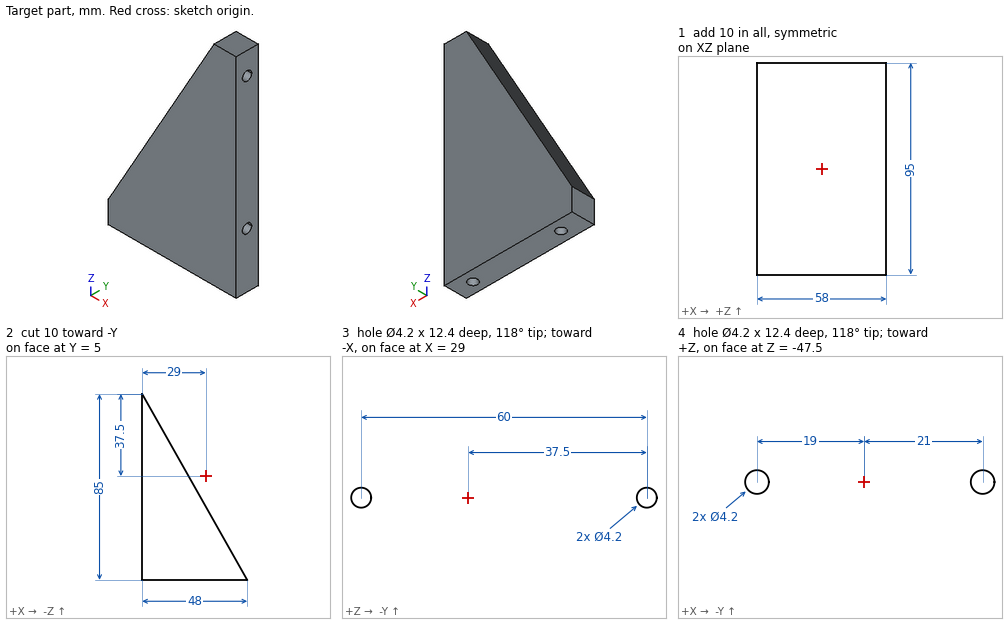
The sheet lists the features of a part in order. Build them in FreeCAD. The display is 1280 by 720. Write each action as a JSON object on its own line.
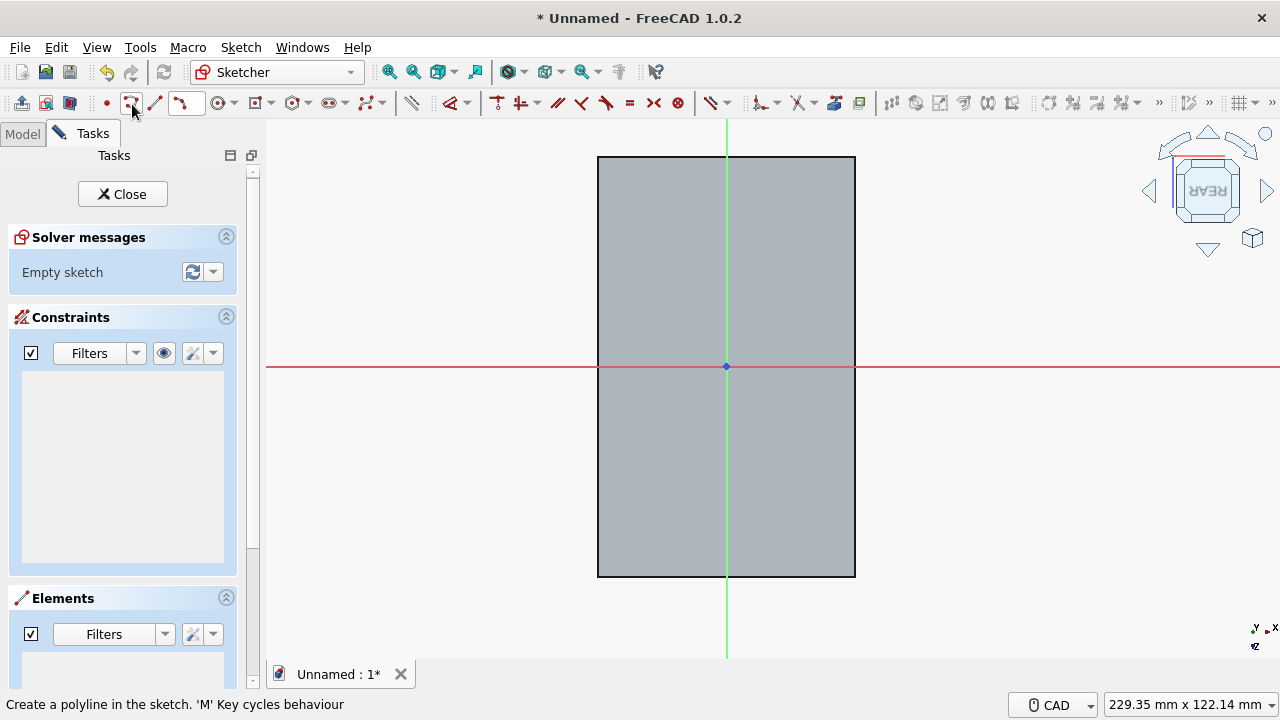
{"action": "left_click", "coordinate": [598, 201]}
{"action": "left_click", "coordinate": [598, 577]}
{"action": "left_click", "coordinate": [811, 577]}
{"action": "left_click", "coordinate": [598, 202]}
{"action": "key", "text": "Escape"}
{"action": "key", "text": "Escape"}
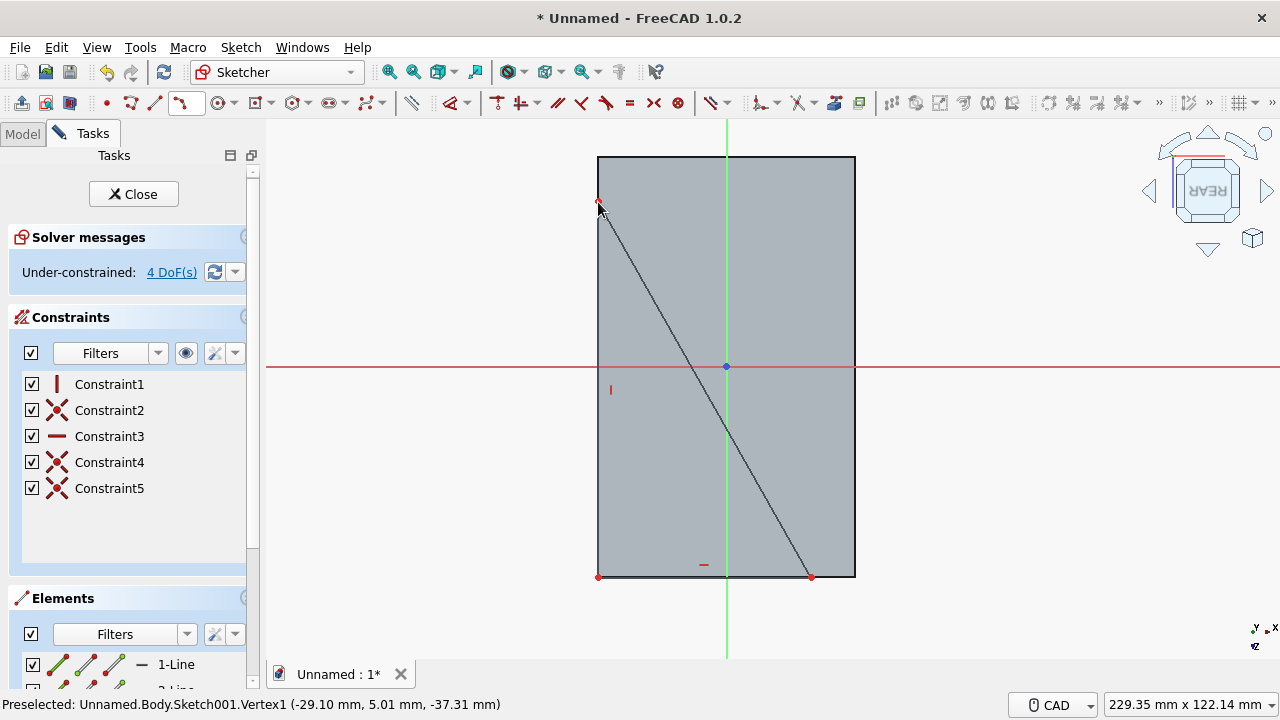
{"action": "left_click", "coordinate": [450, 104]}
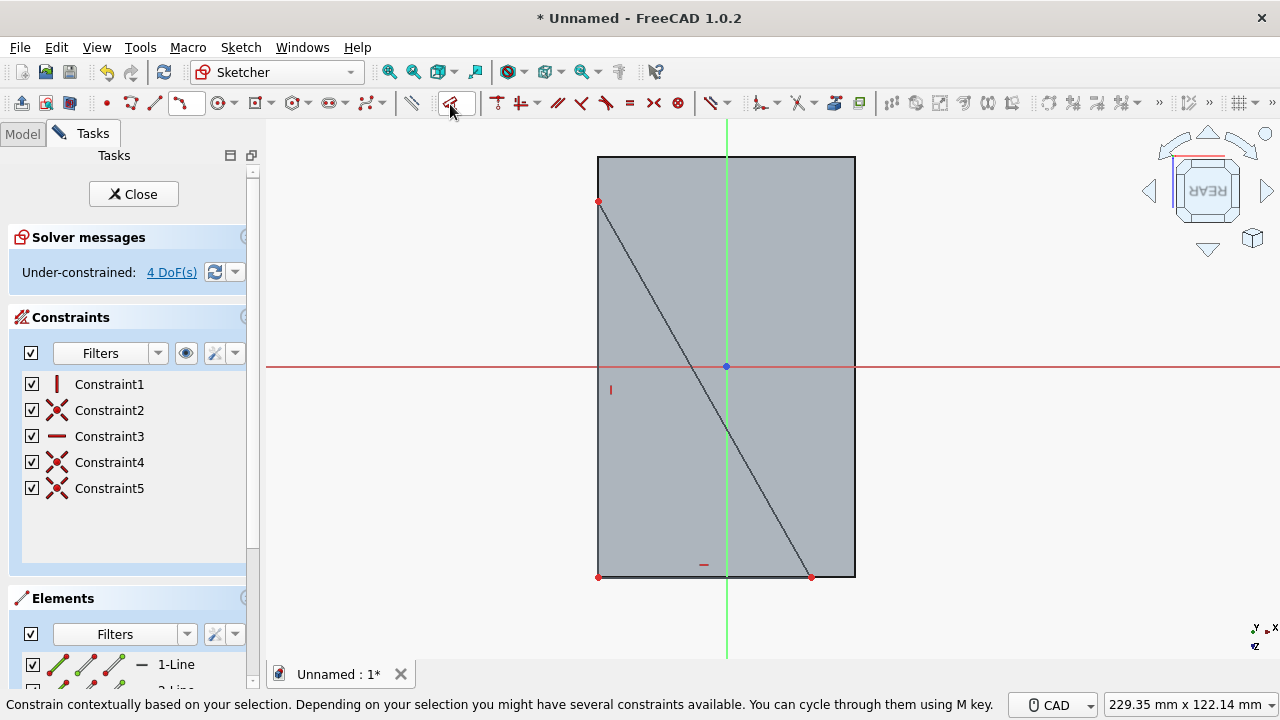
{"action": "left_click", "coordinate": [598, 315]}
{"action": "left_click", "coordinate": [564, 390]}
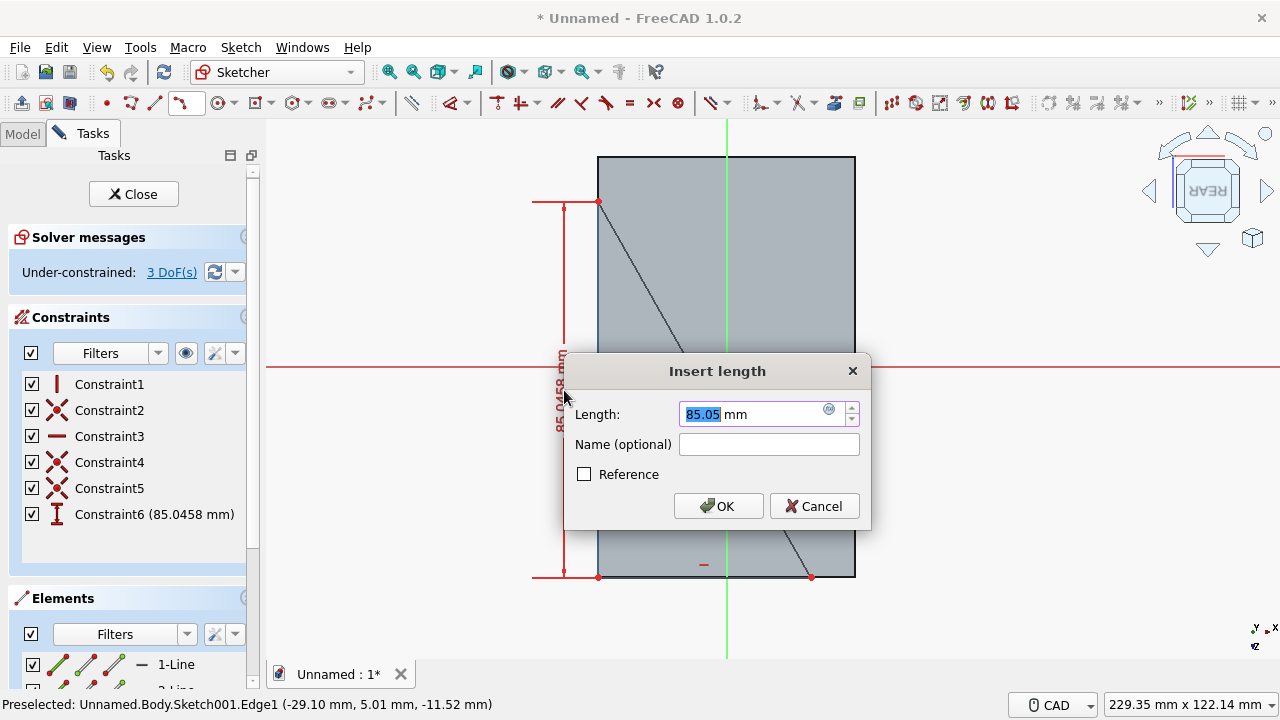
{"action": "type", "text": "85"}
{"action": "key", "text": "Return"}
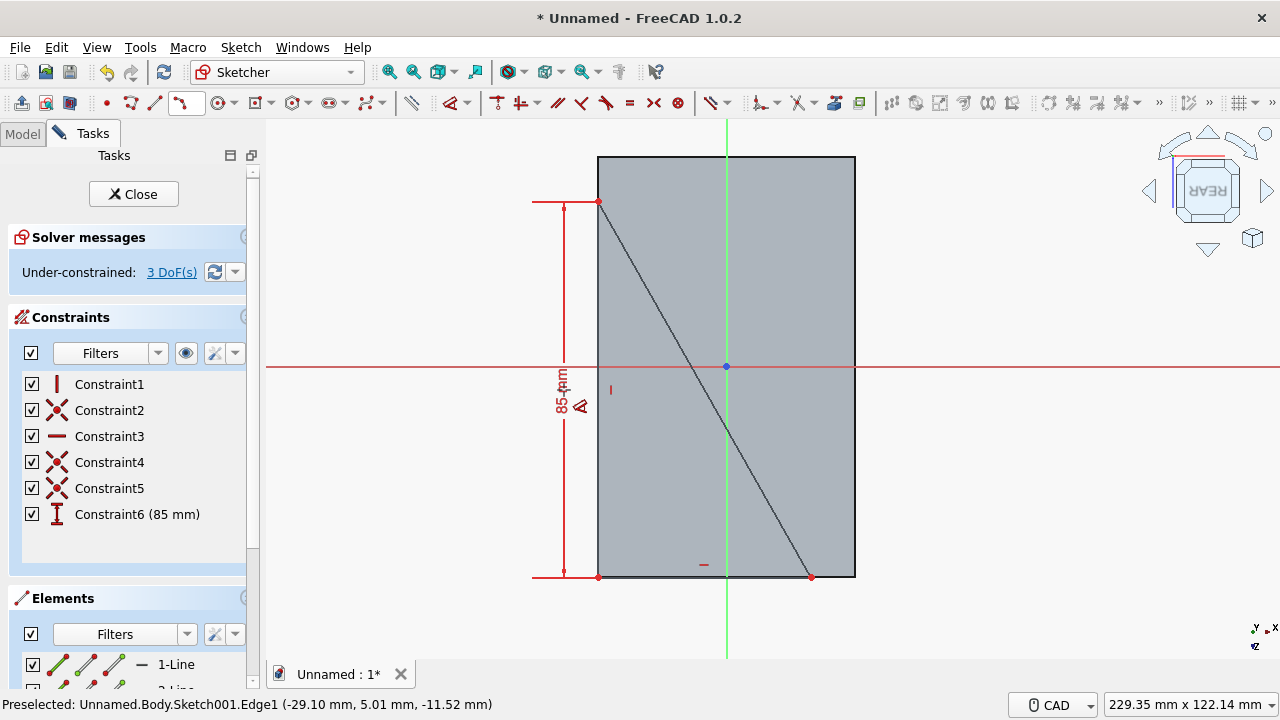
{"action": "left_click", "coordinate": [662, 578]}
{"action": "left_click", "coordinate": [705, 612]}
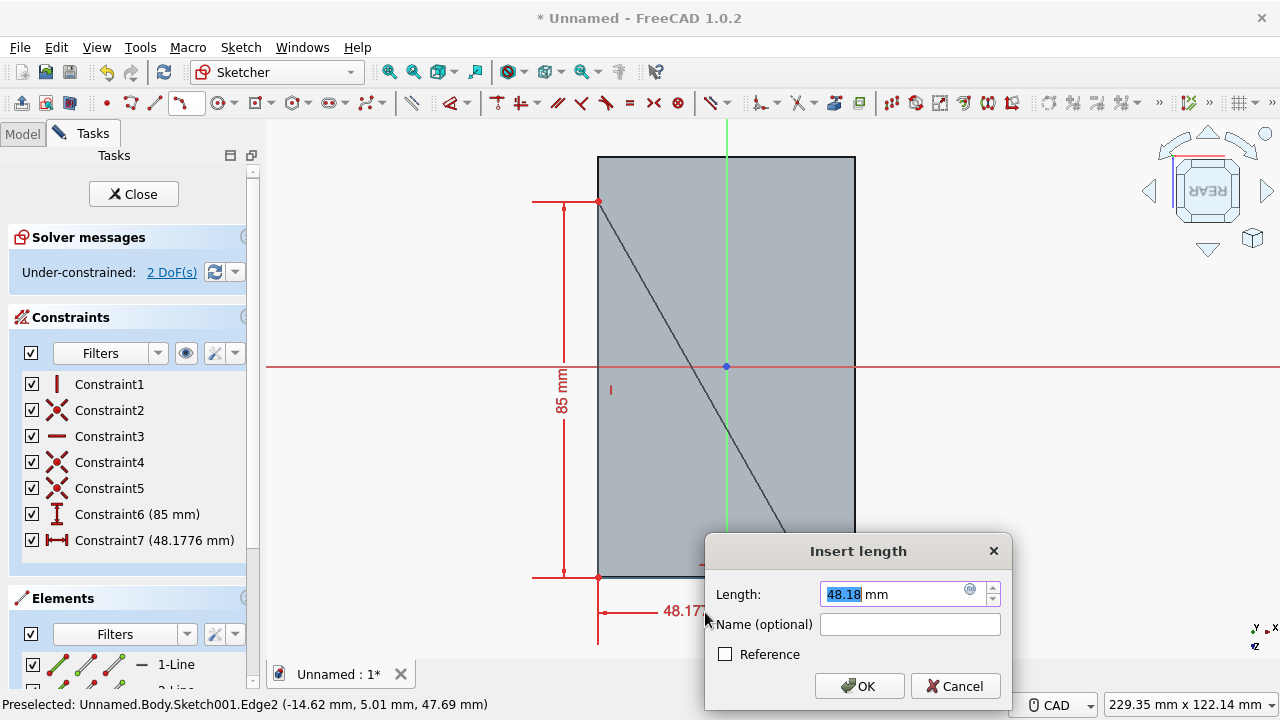
{"action": "type", "text": "48"}
{"action": "key", "text": "Return"}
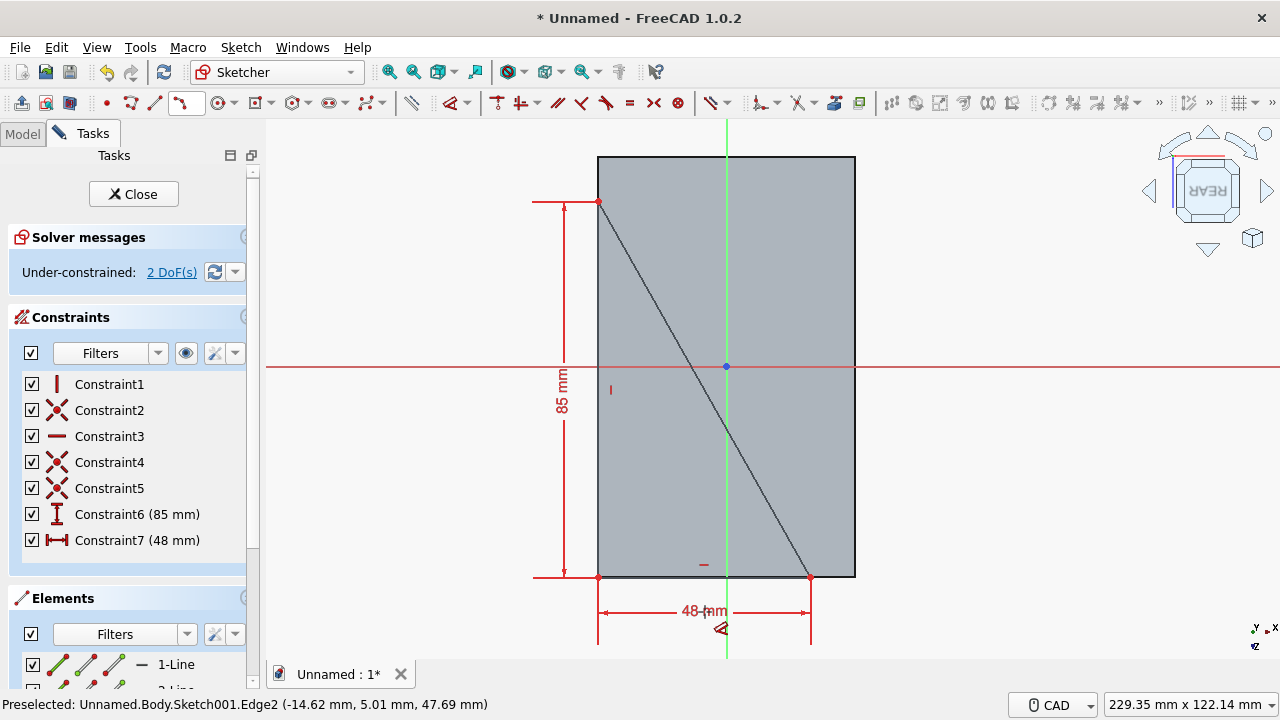
{"action": "left_click", "coordinate": [598, 202]}
{"action": "left_click", "coordinate": [662, 168]}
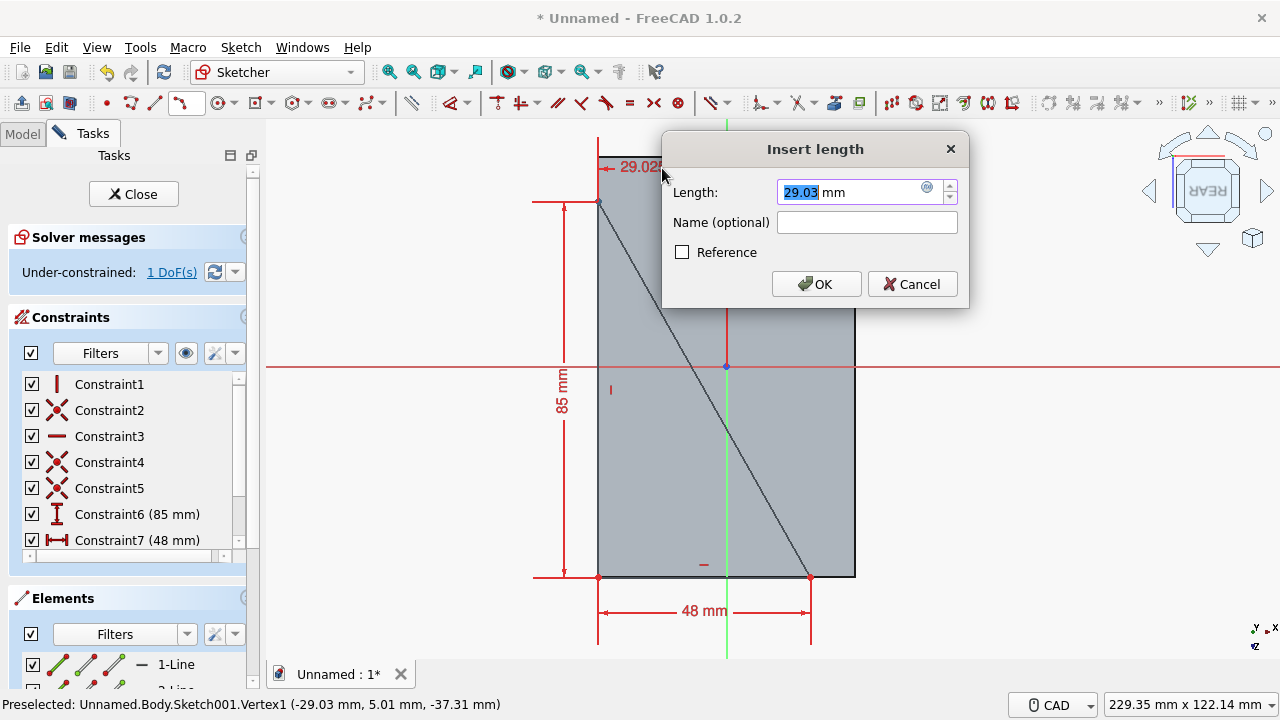
{"action": "type", "text": "29"}
{"action": "key", "text": "Return"}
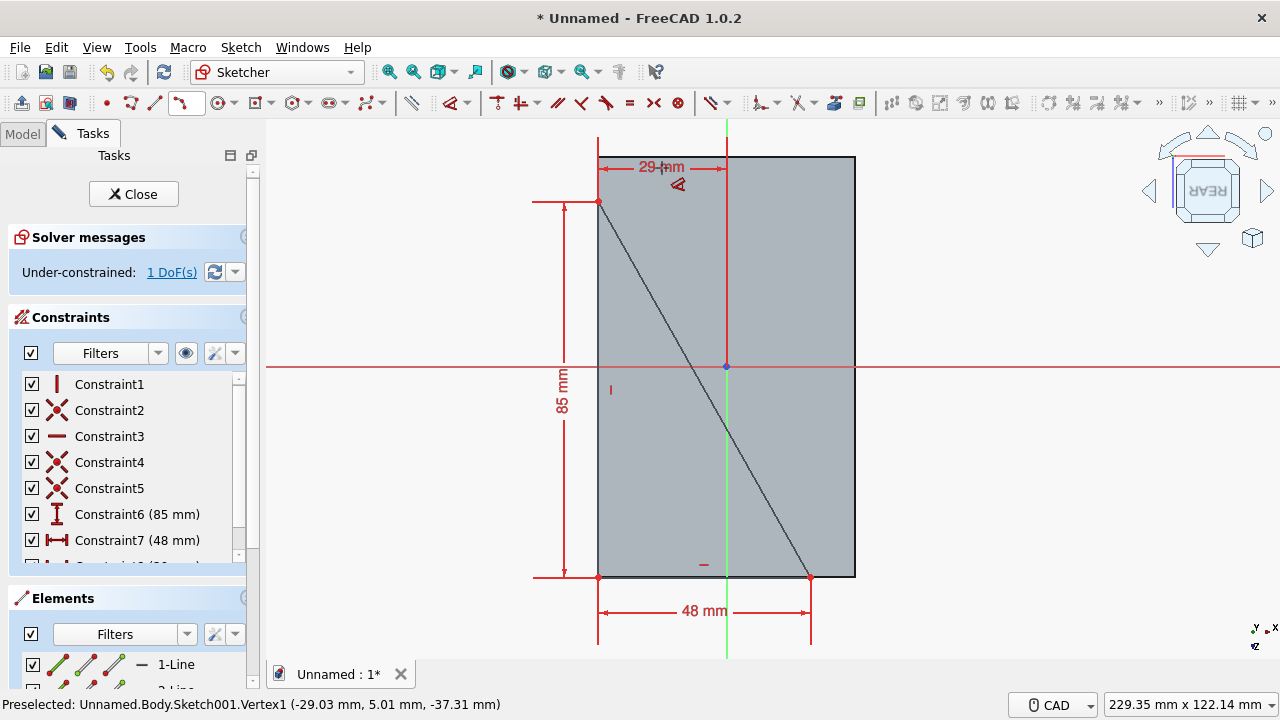
{"action": "left_click", "coordinate": [598, 202]}
{"action": "left_click", "coordinate": [564, 284]}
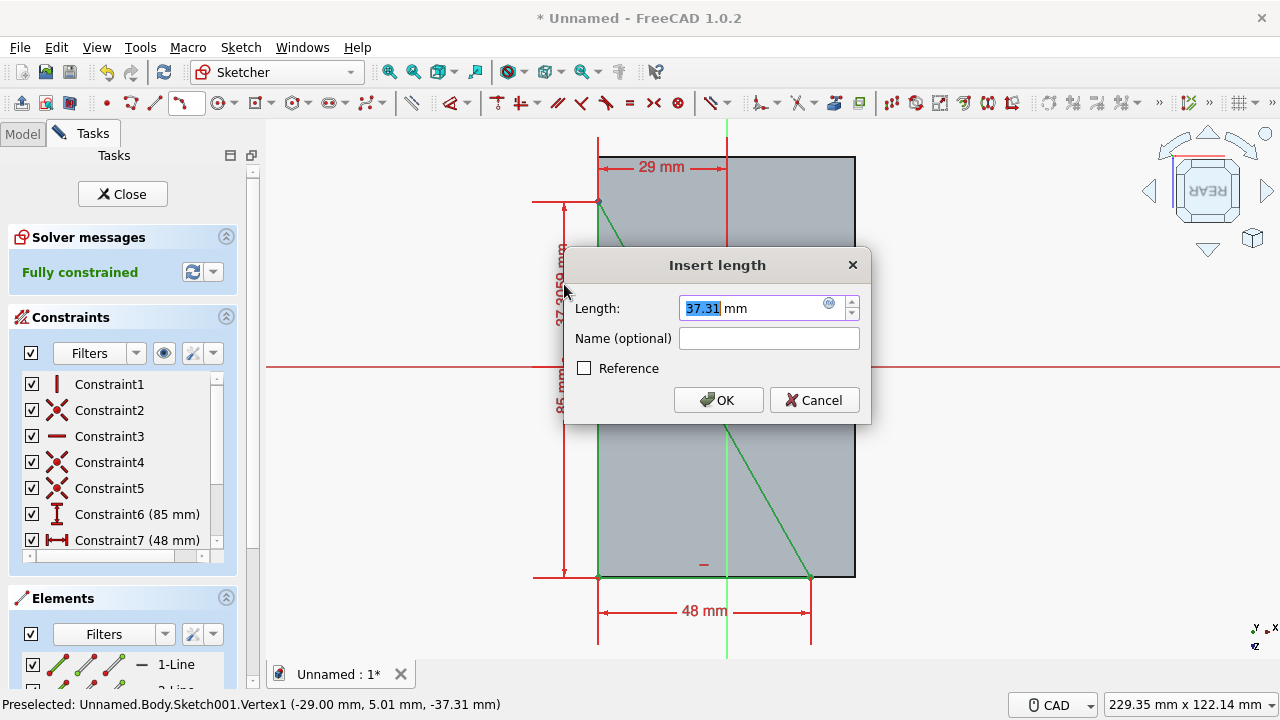
{"action": "type", "text": "37.5"}
{"action": "key", "text": "Return"}
{"action": "key", "text": "Escape"}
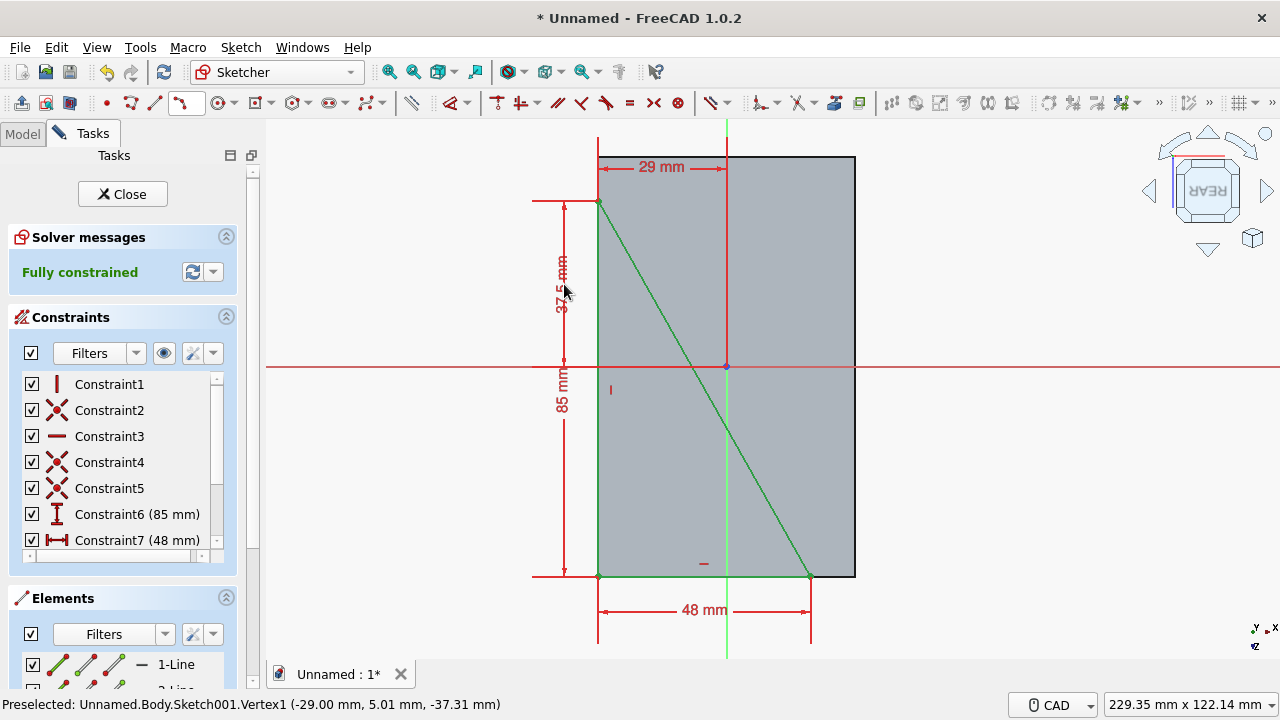
{"action": "left_click", "coordinate": [123, 194]}